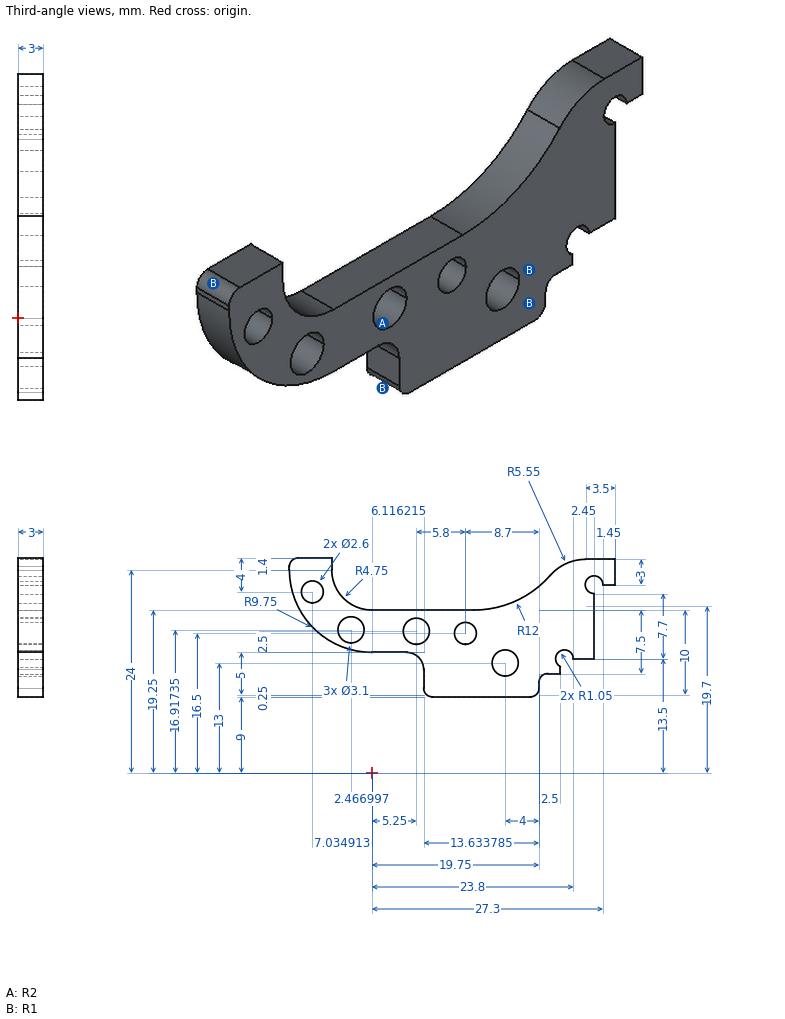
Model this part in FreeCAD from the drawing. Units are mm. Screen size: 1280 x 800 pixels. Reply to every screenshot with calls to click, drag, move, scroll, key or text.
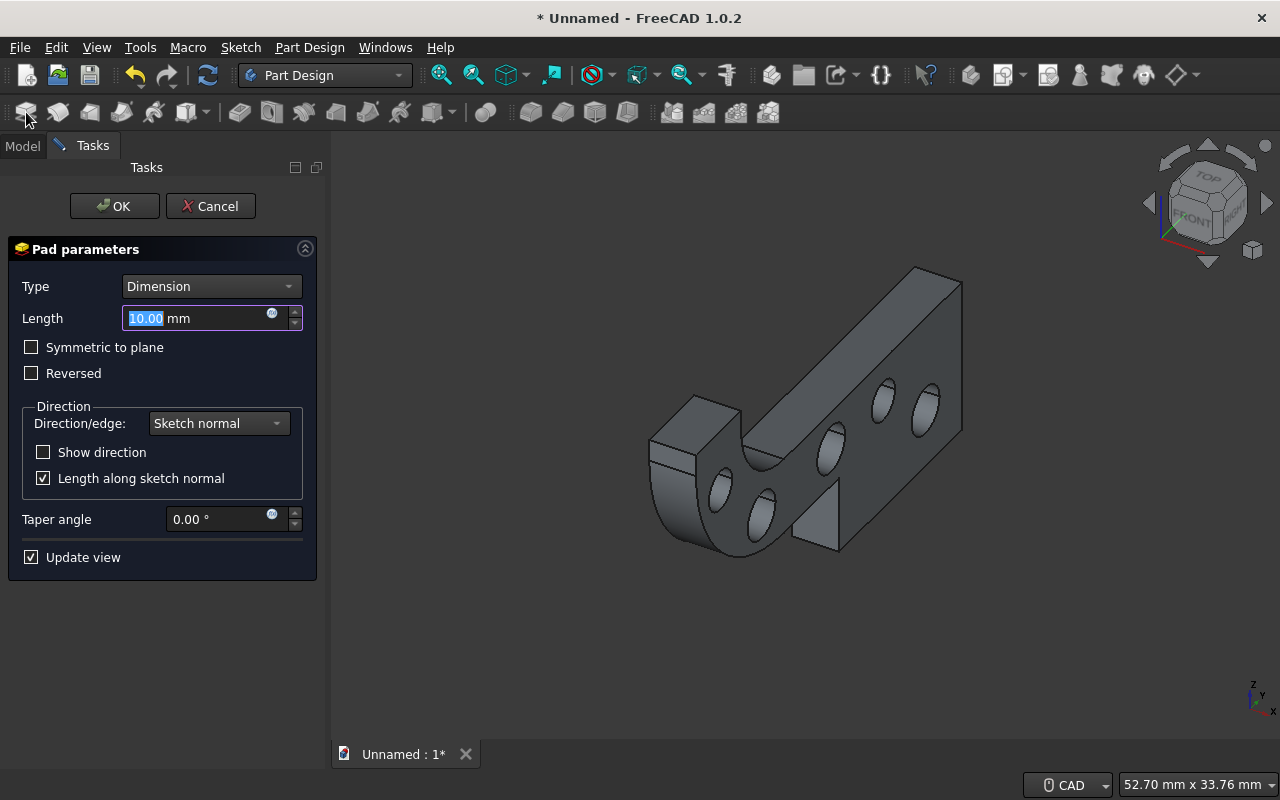
text(3)
key(Tab)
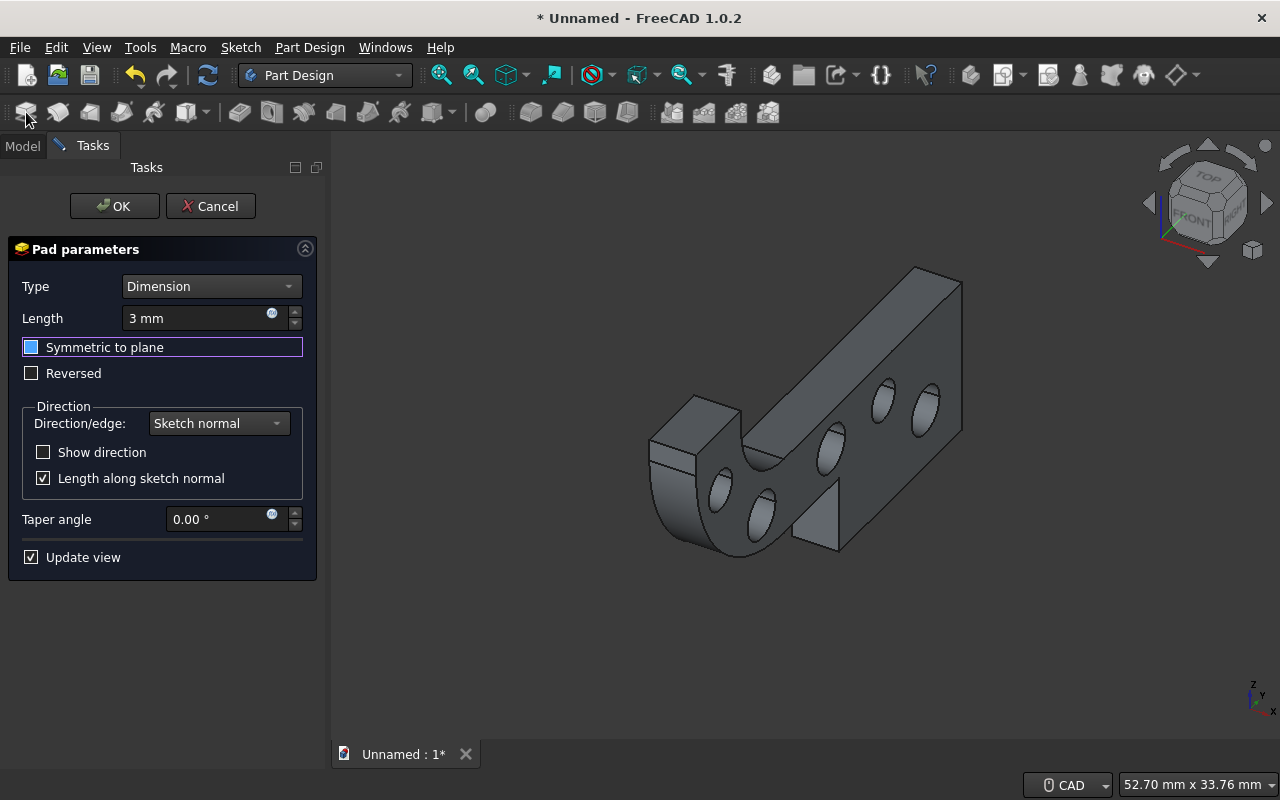
click(30, 373)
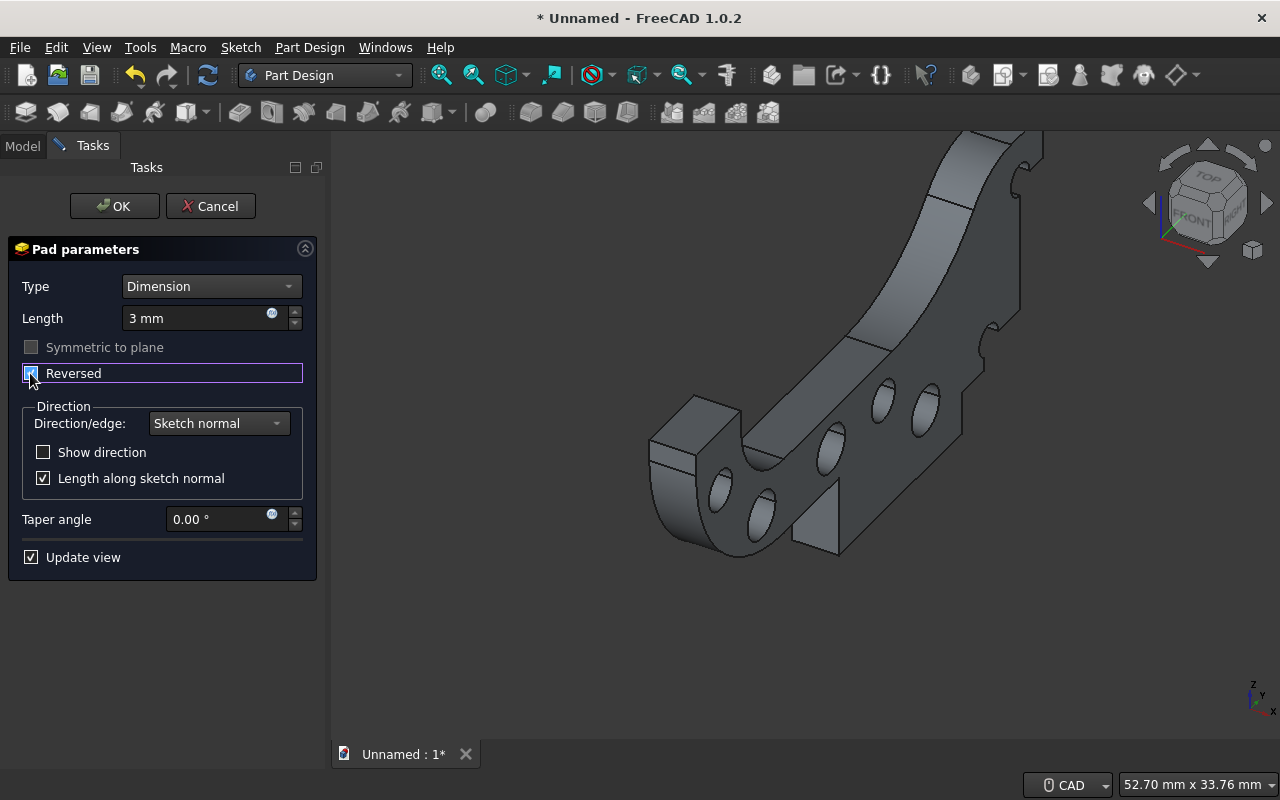
click(115, 206)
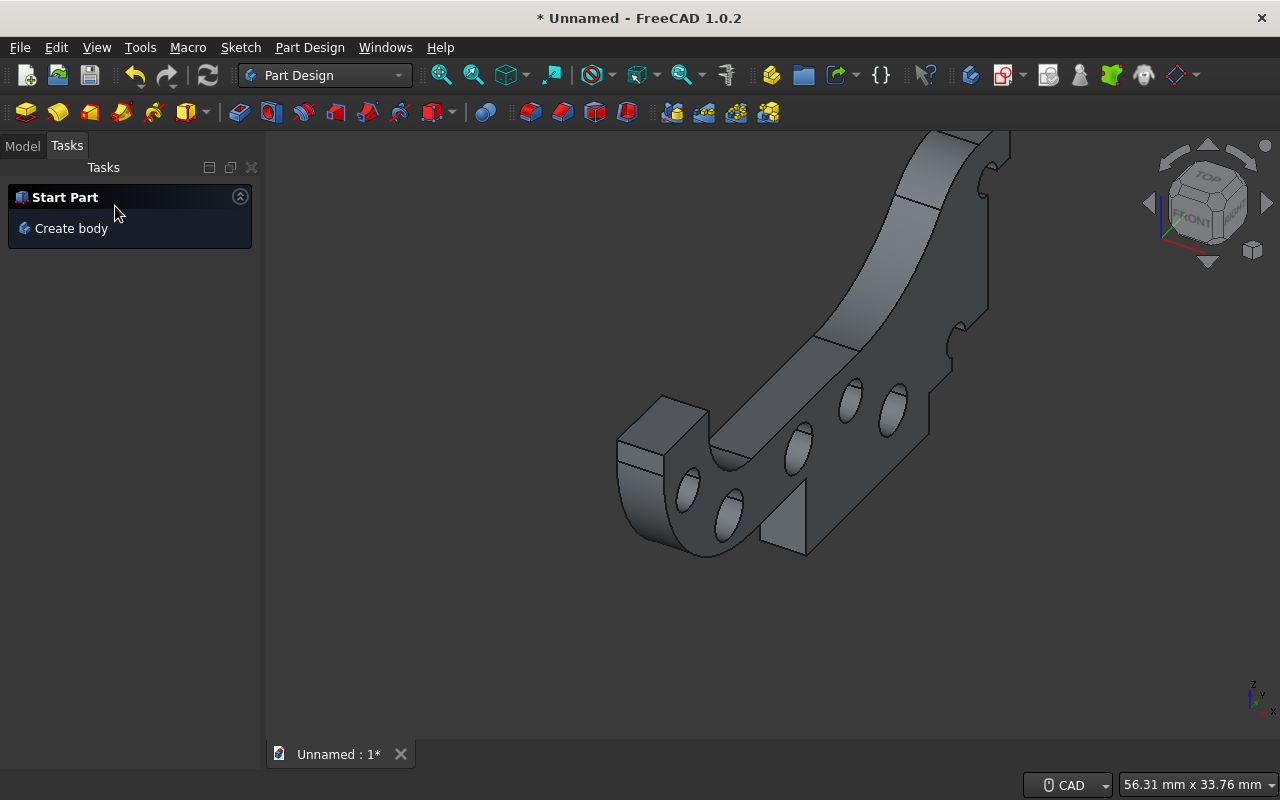
key(v)
key(f)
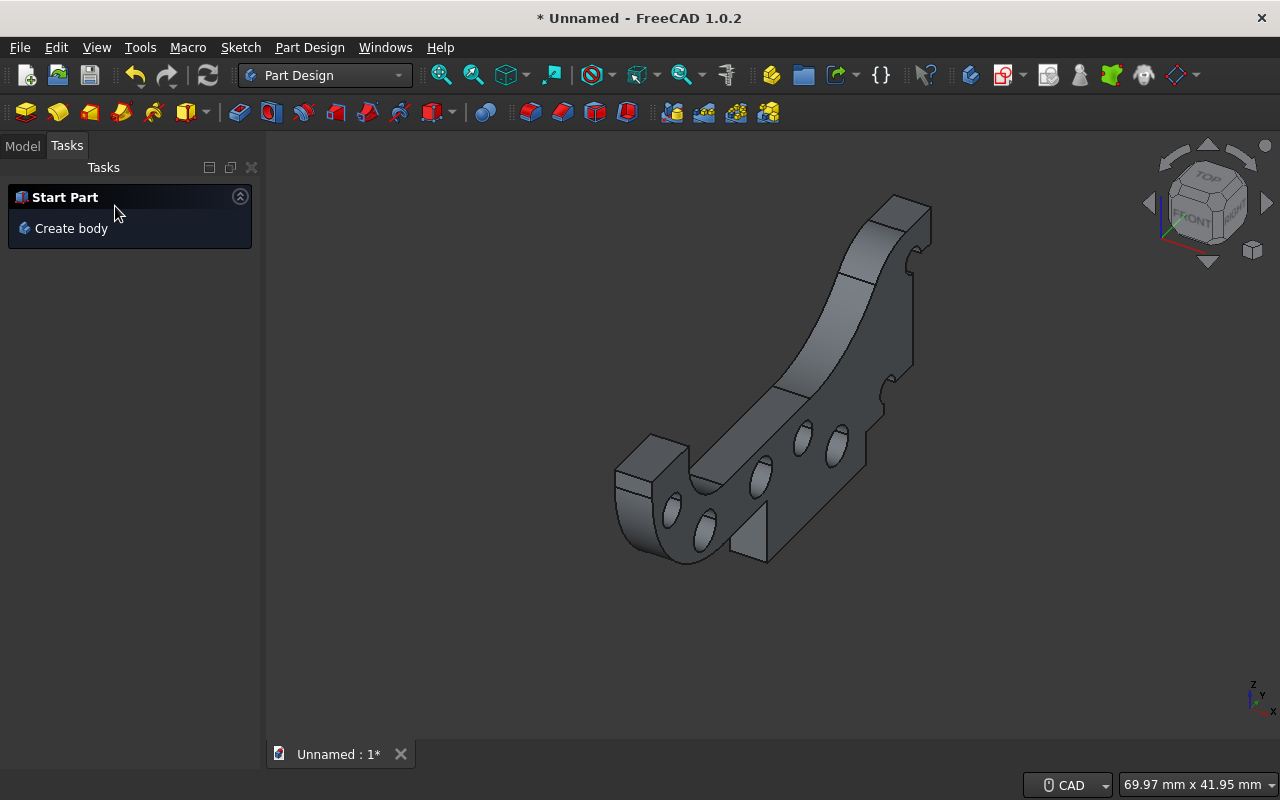
key(0)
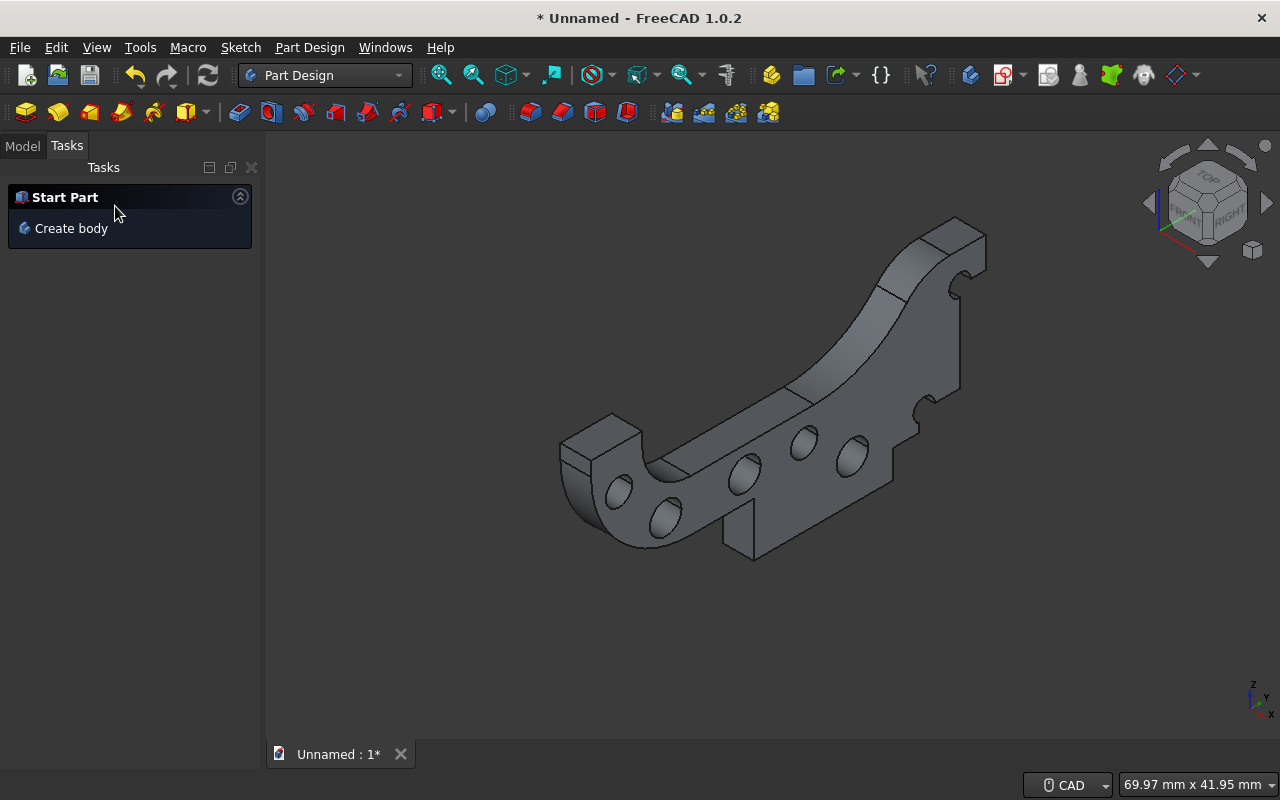
key(2)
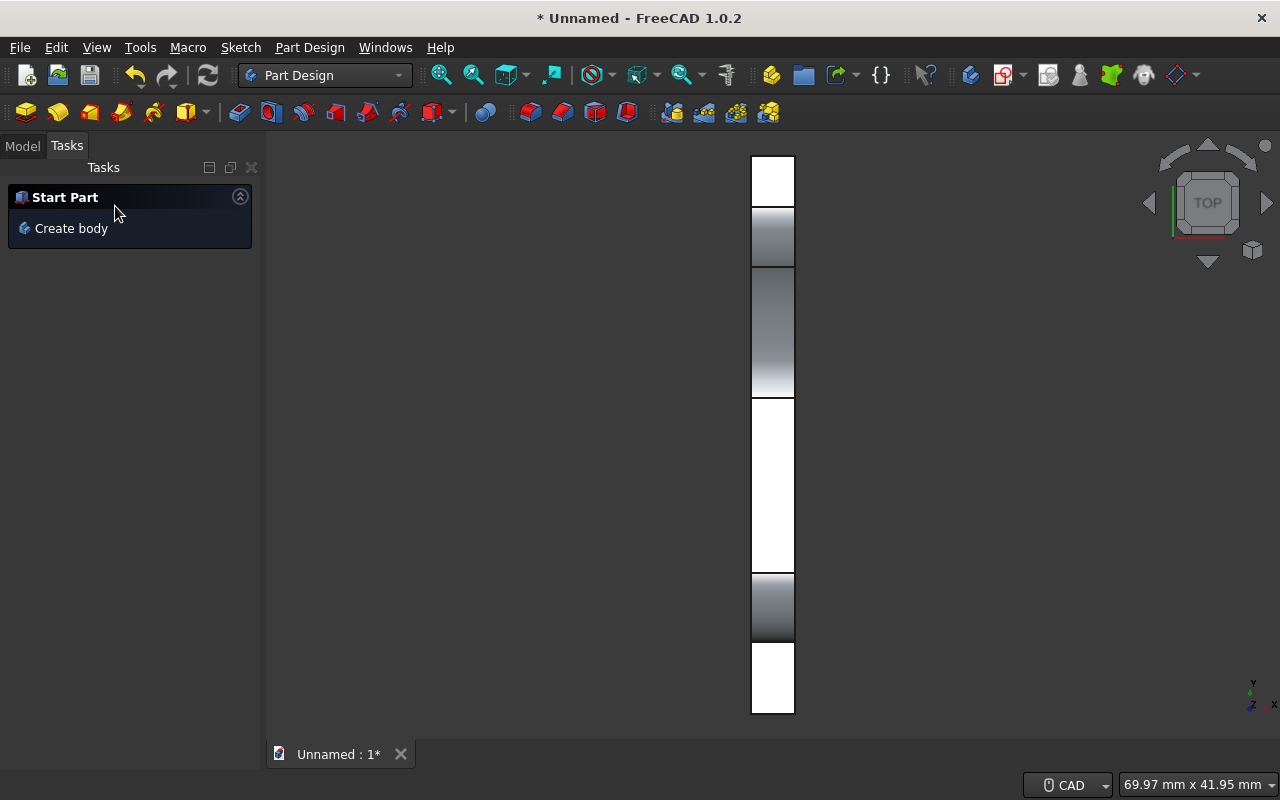
key(1)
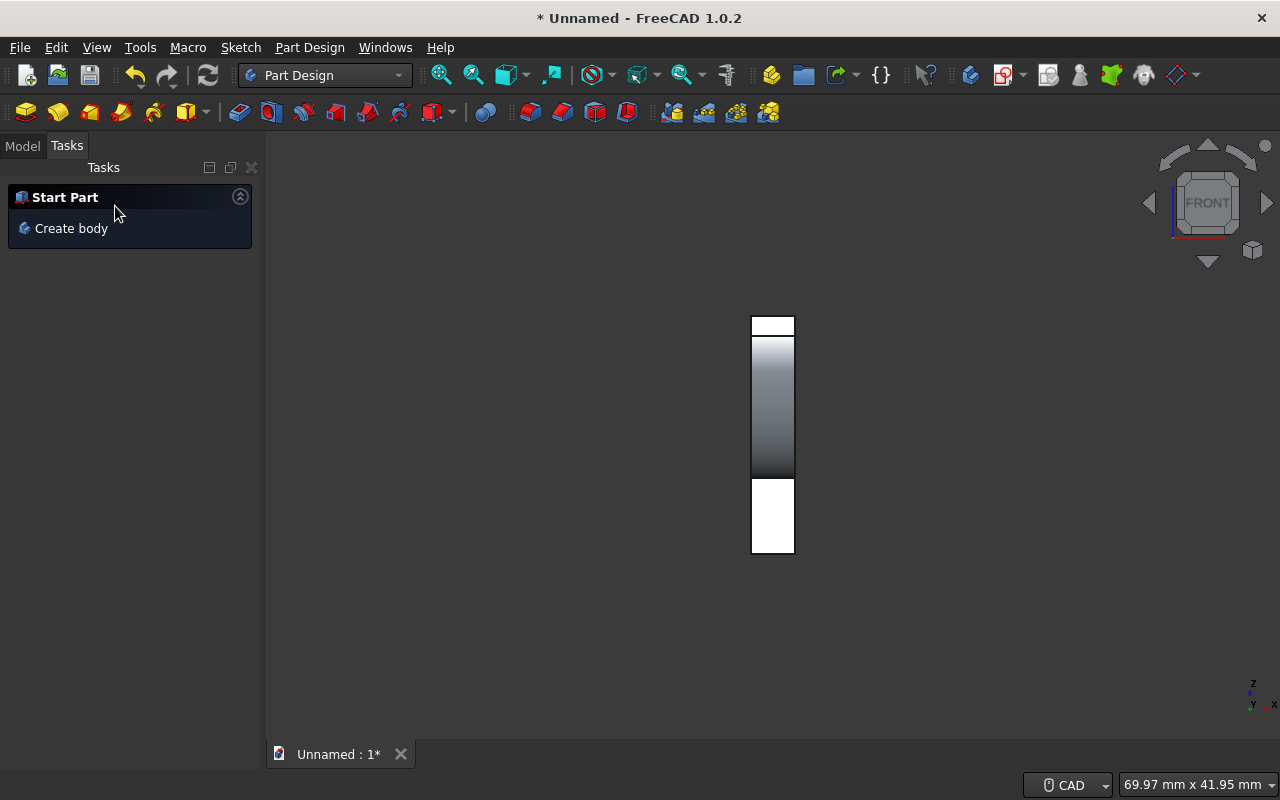
key(v)
key(f)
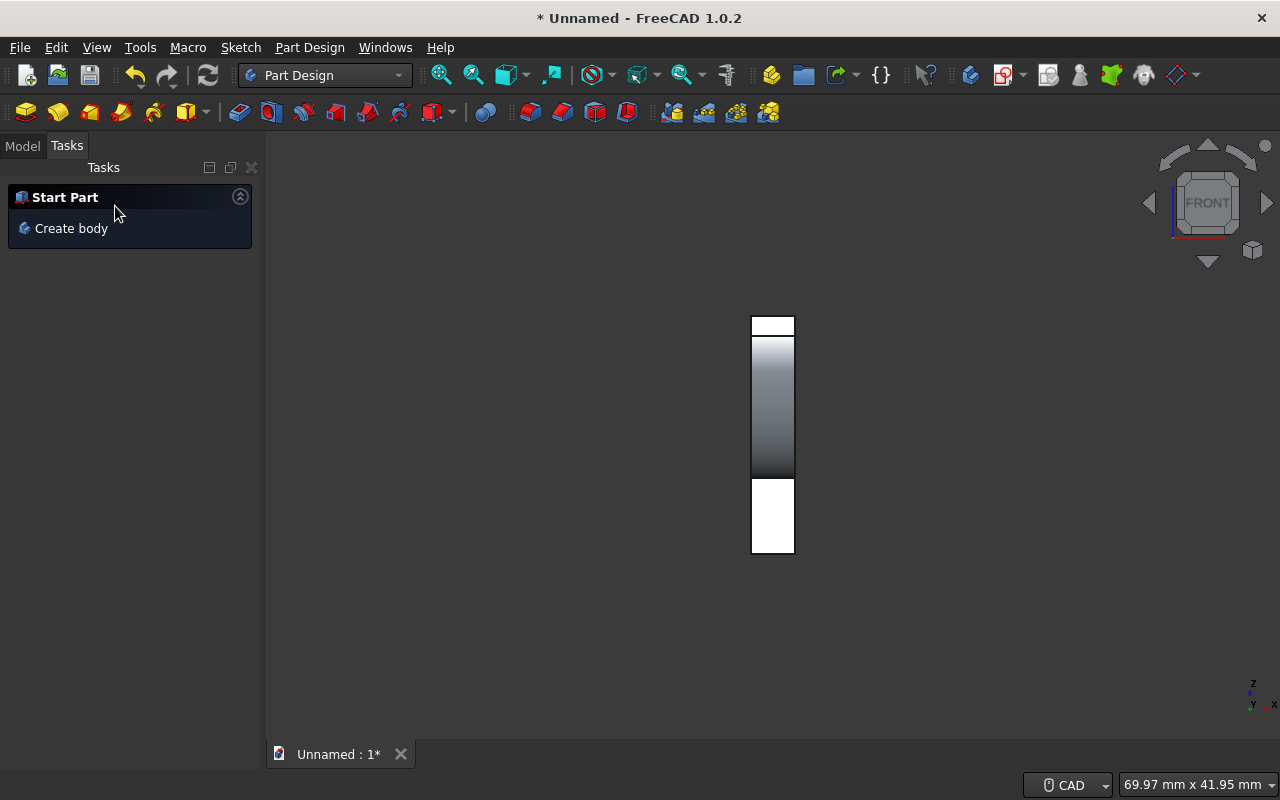
key(3)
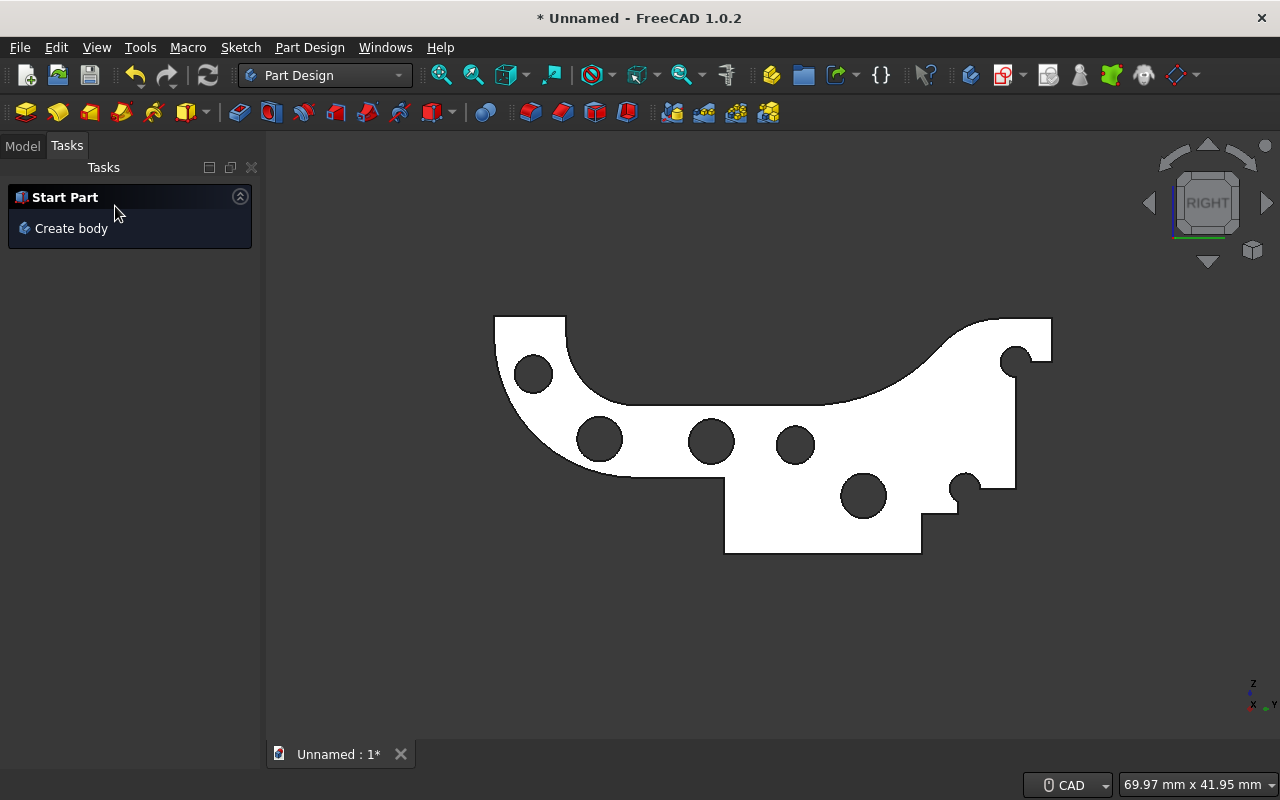
key(5)